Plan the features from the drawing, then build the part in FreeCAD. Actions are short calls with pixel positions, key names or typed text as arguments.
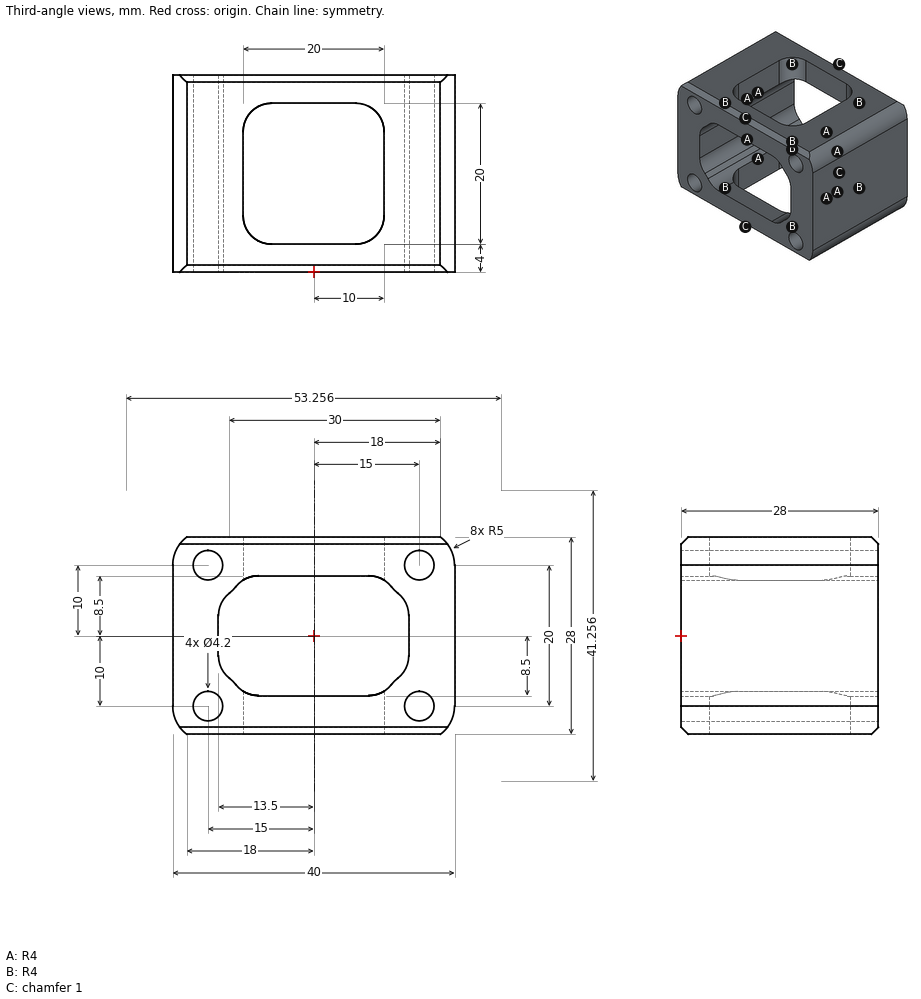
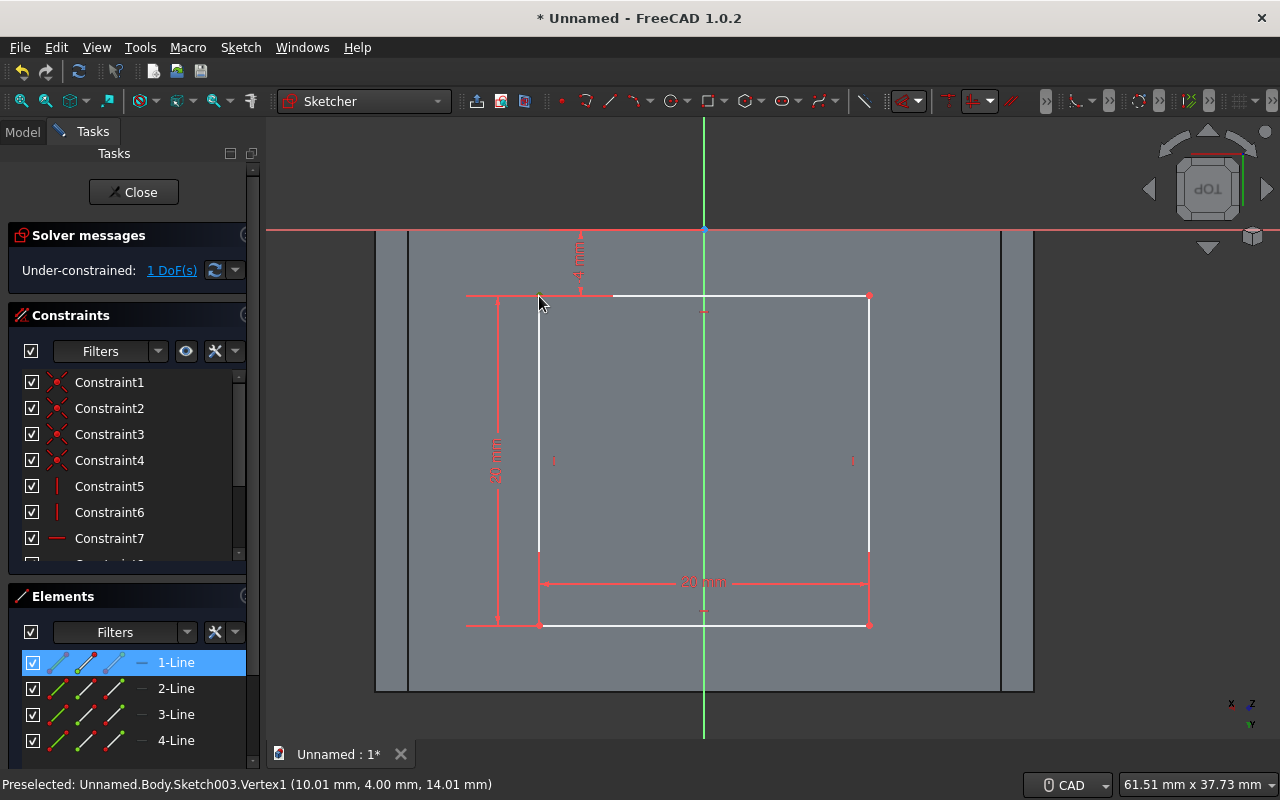
key(l)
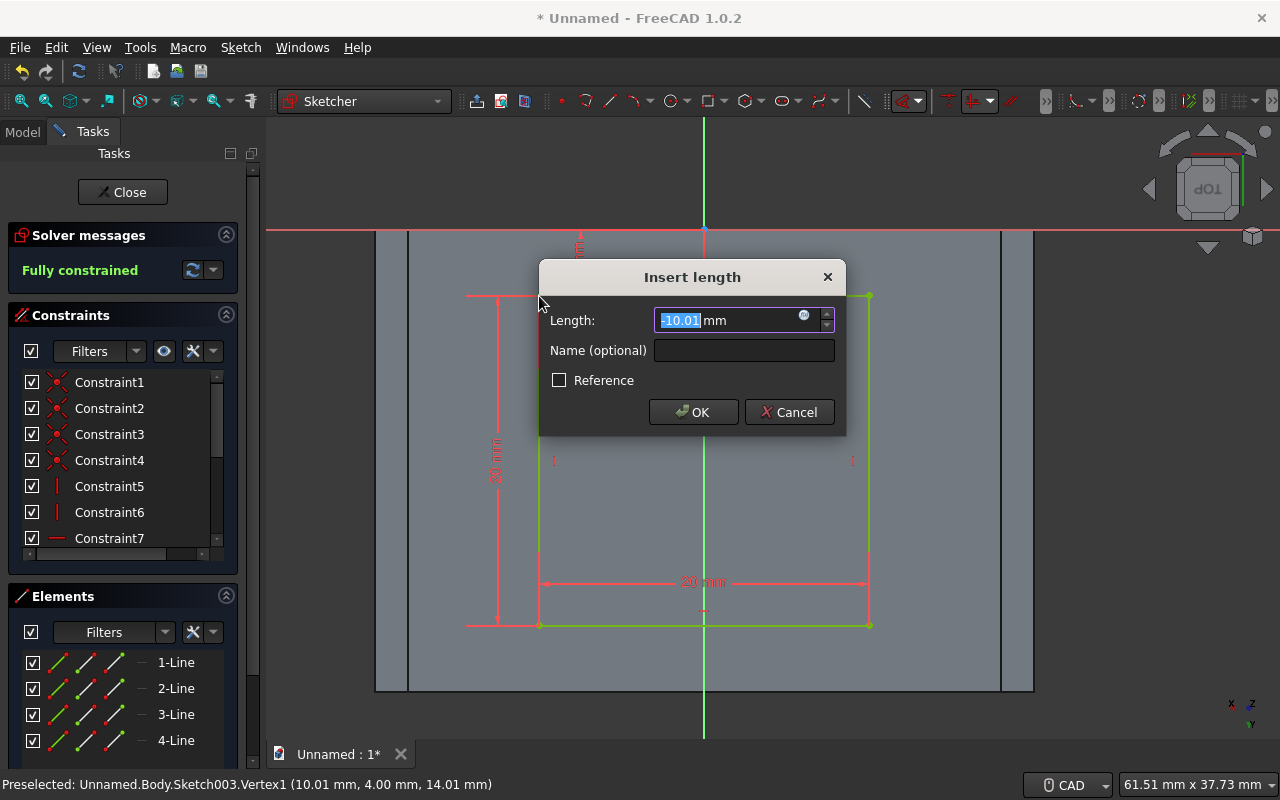
text(-10)
key(Return)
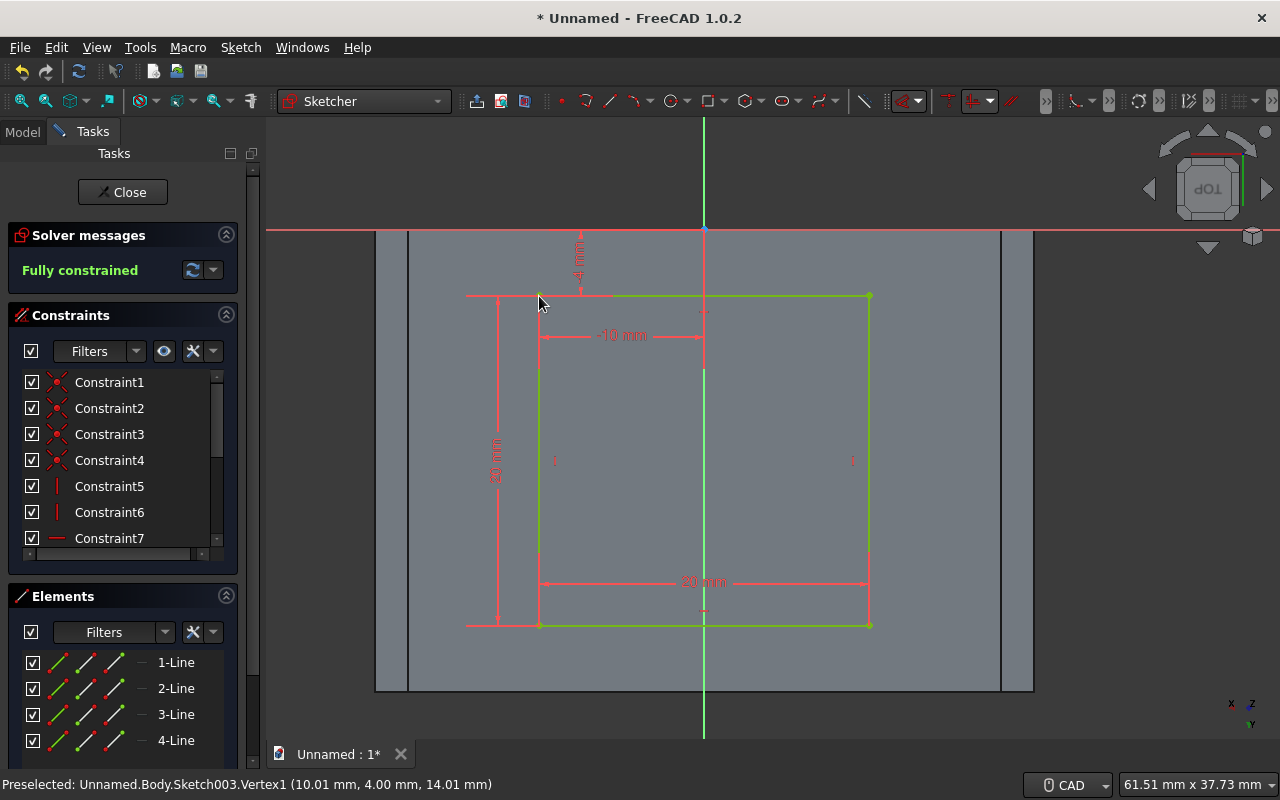
click(123, 192)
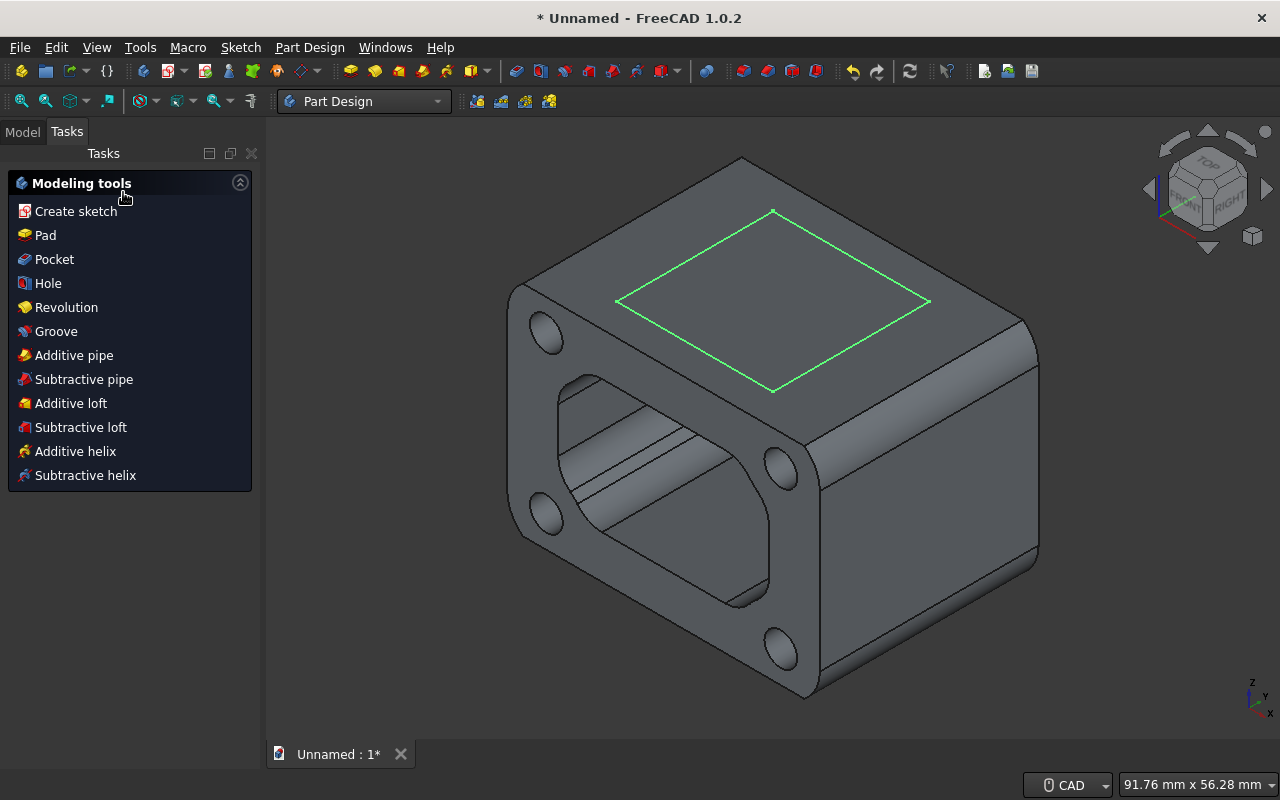
click(518, 72)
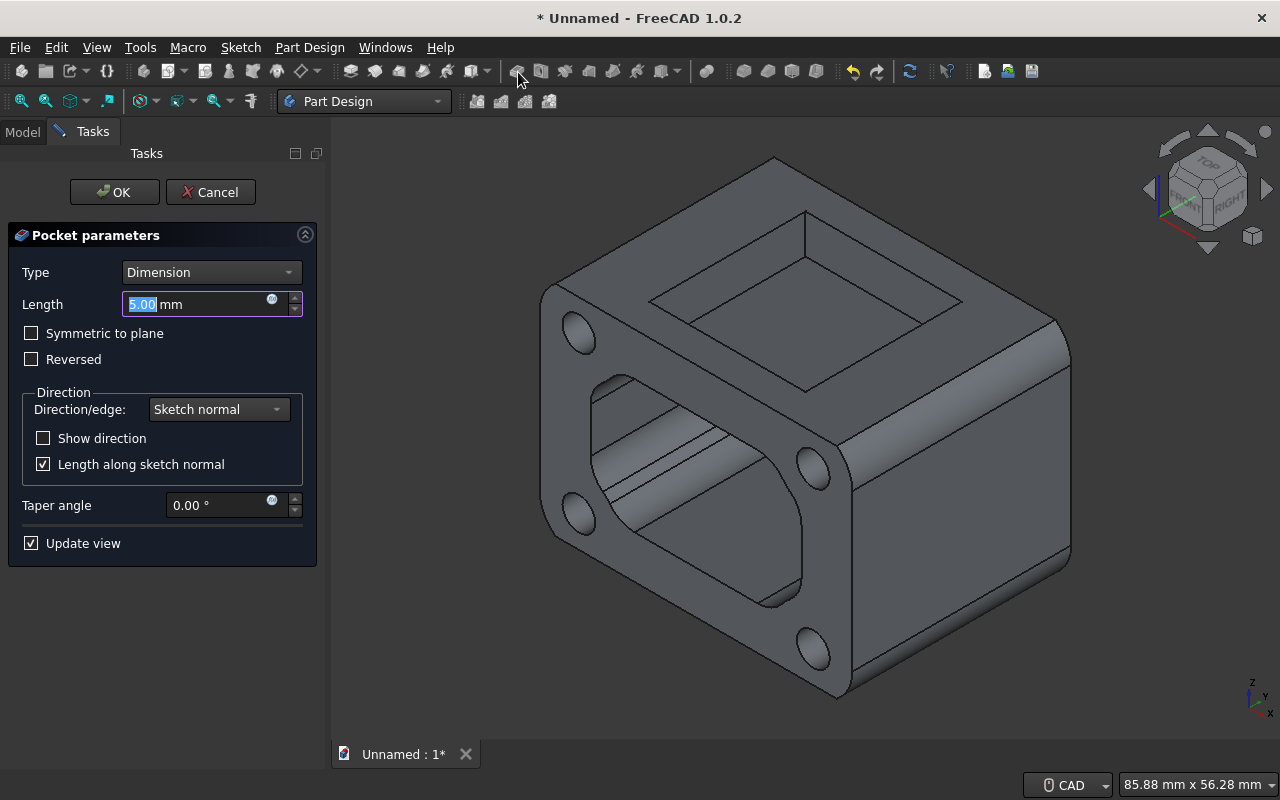
click(212, 272)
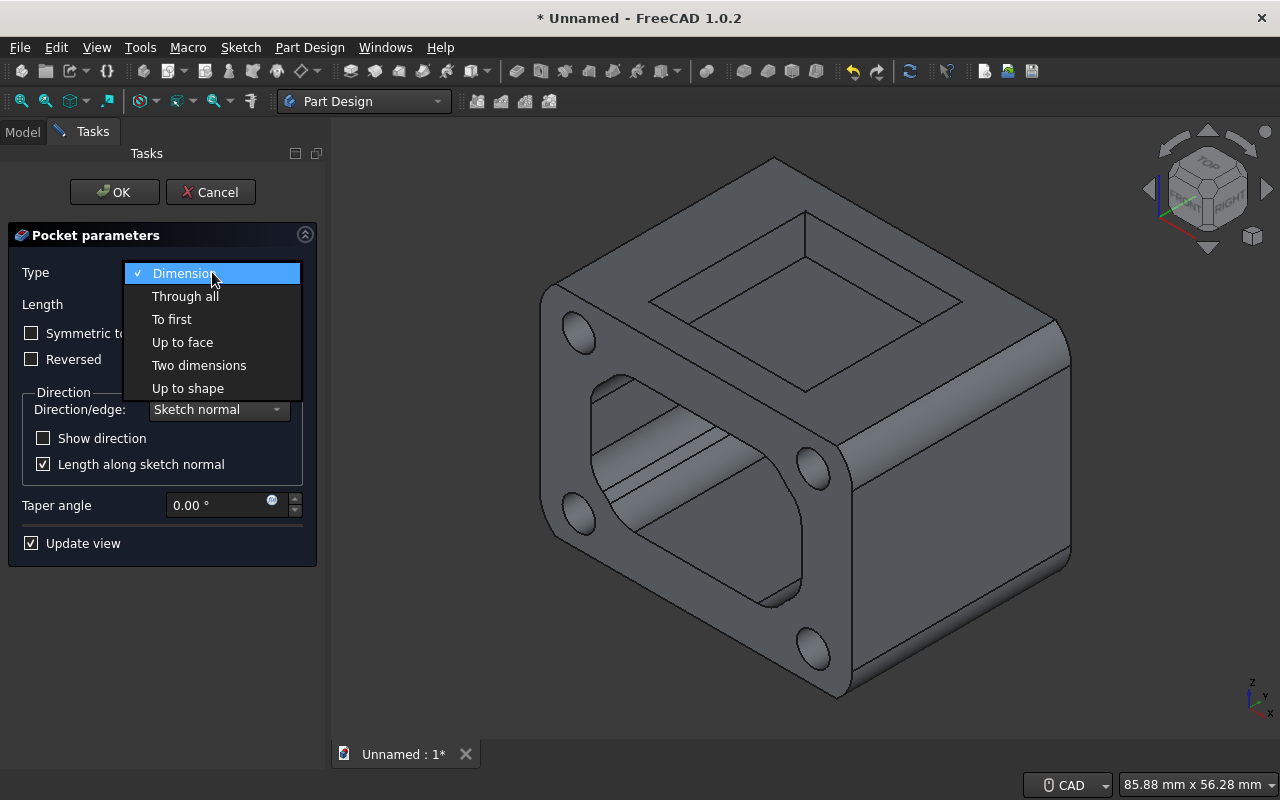
click(212, 296)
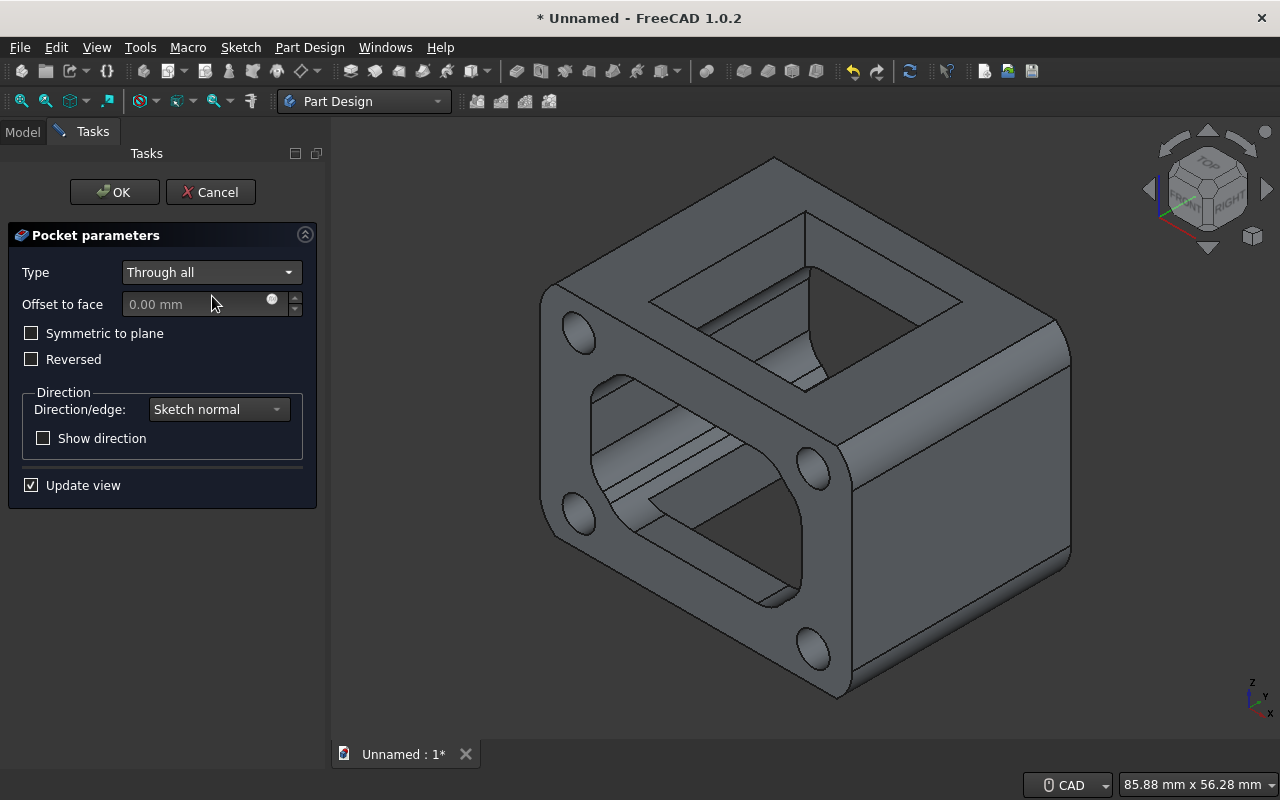
click(115, 192)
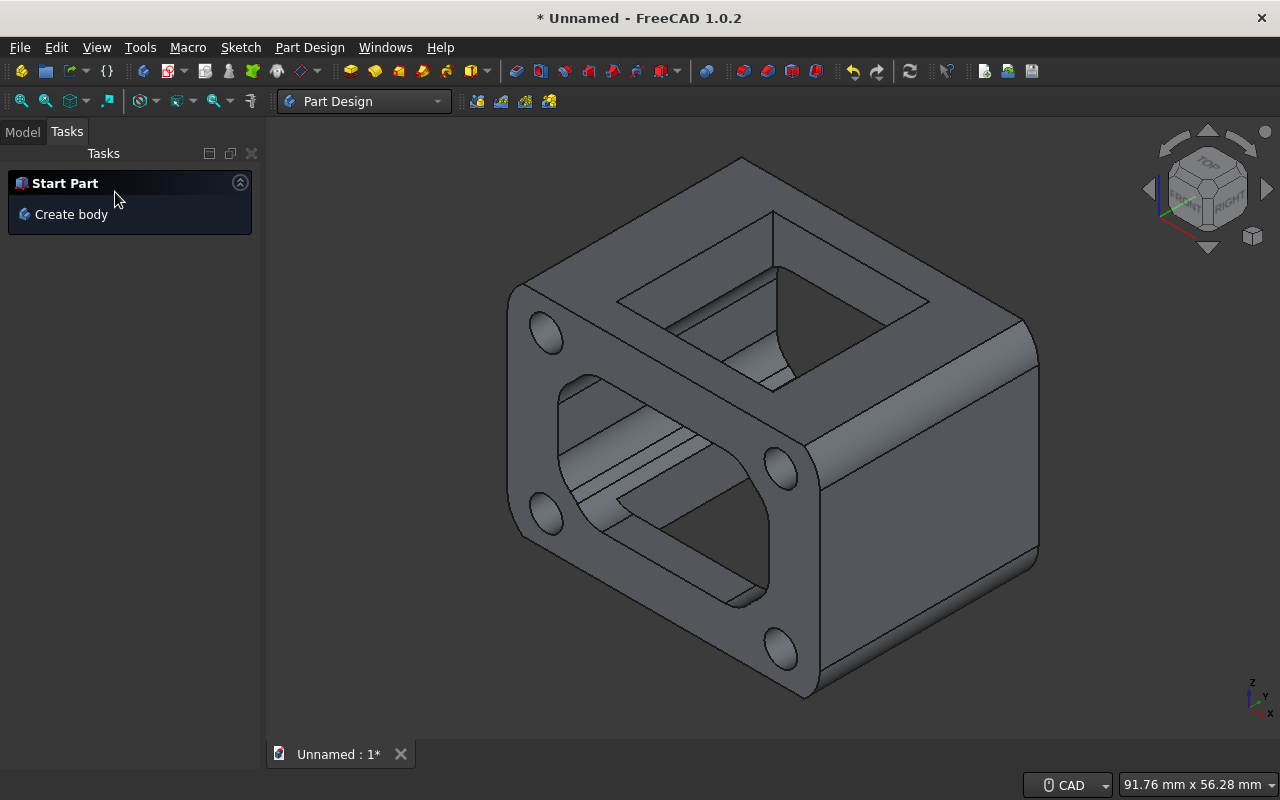
key(2)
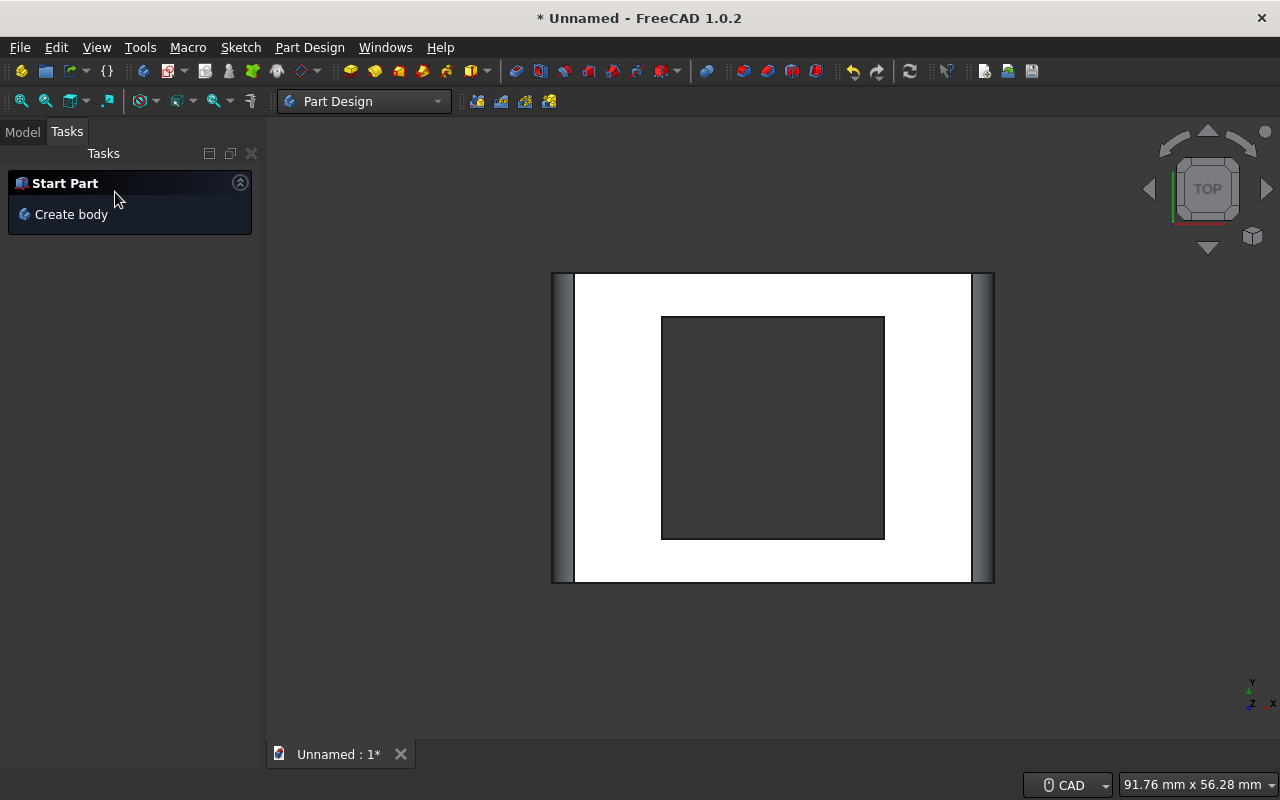
key(0)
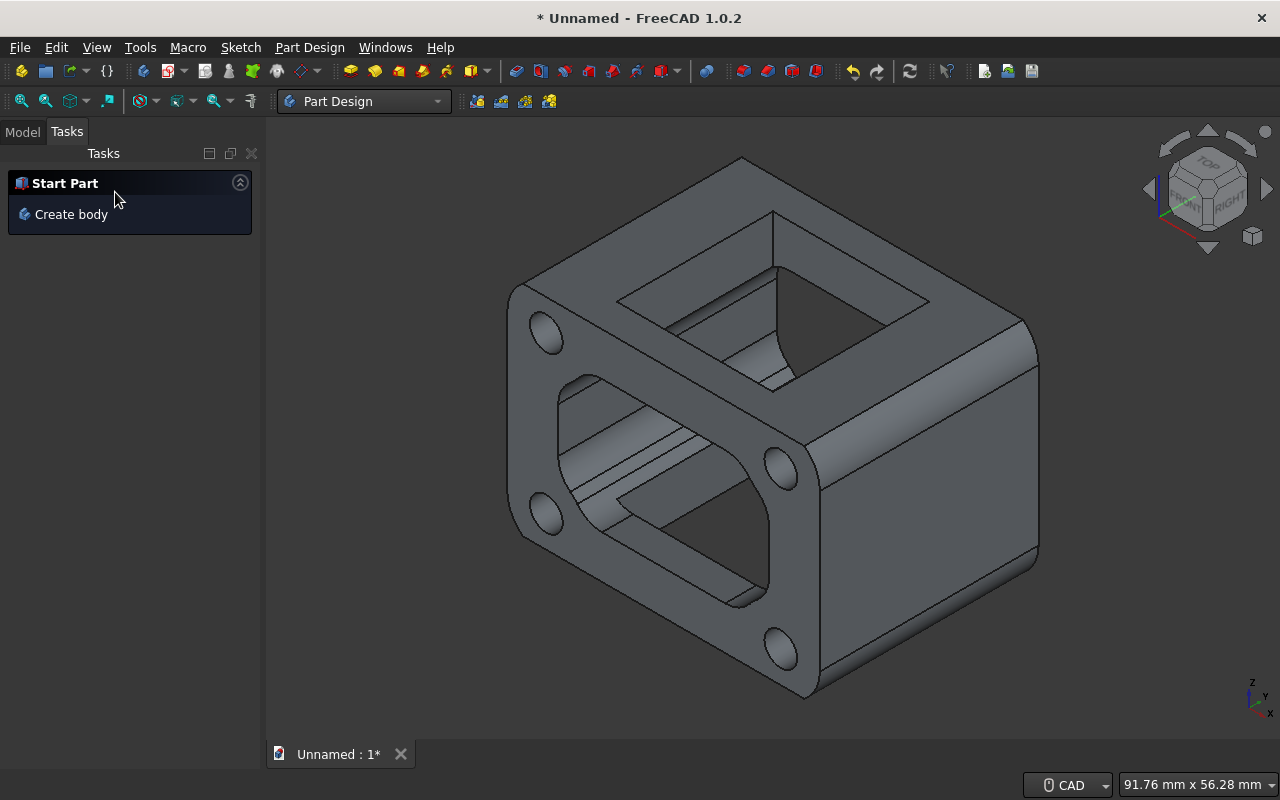
key(1)